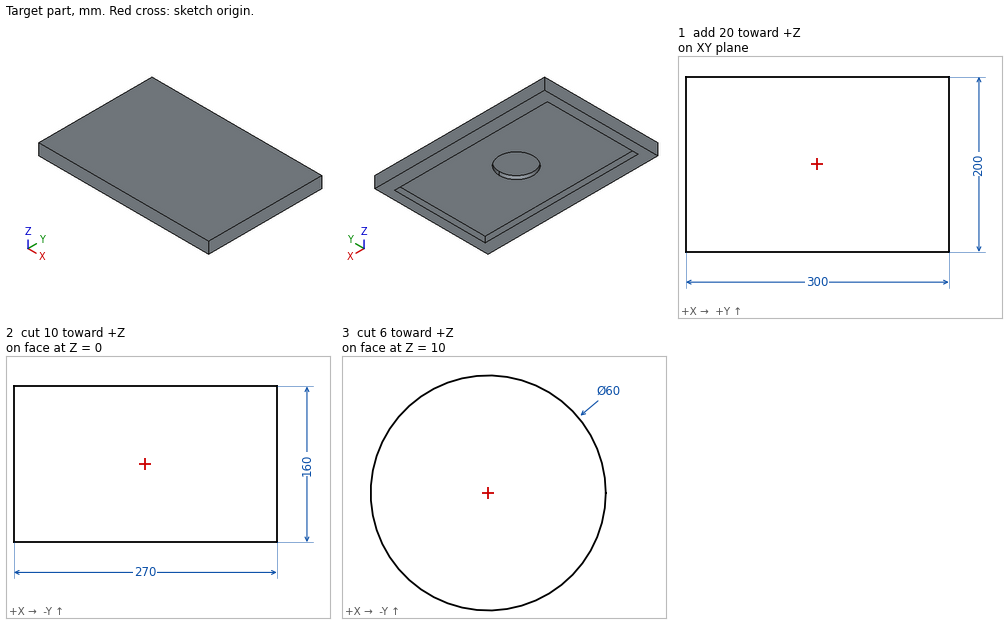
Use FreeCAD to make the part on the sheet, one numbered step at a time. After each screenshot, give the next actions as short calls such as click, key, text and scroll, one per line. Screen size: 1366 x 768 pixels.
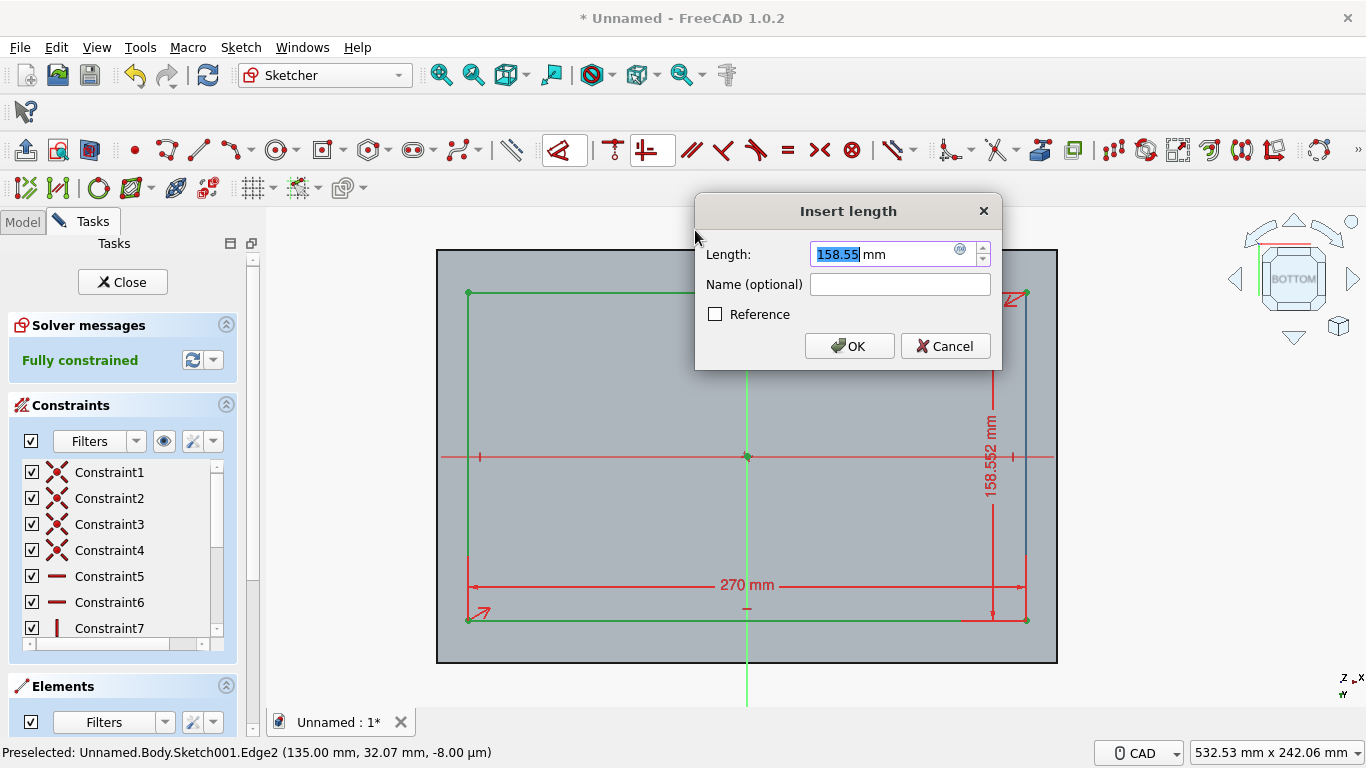
text(160)
key(Return)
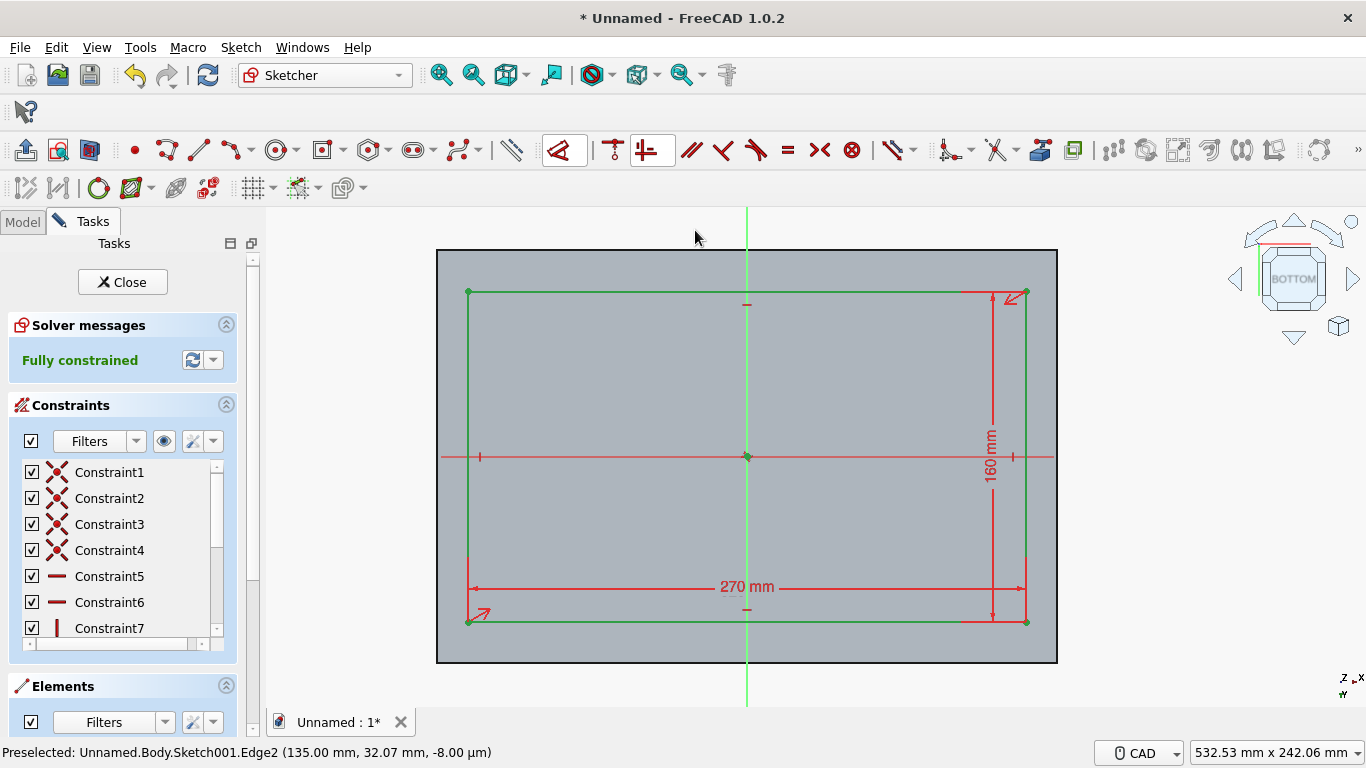
click(123, 282)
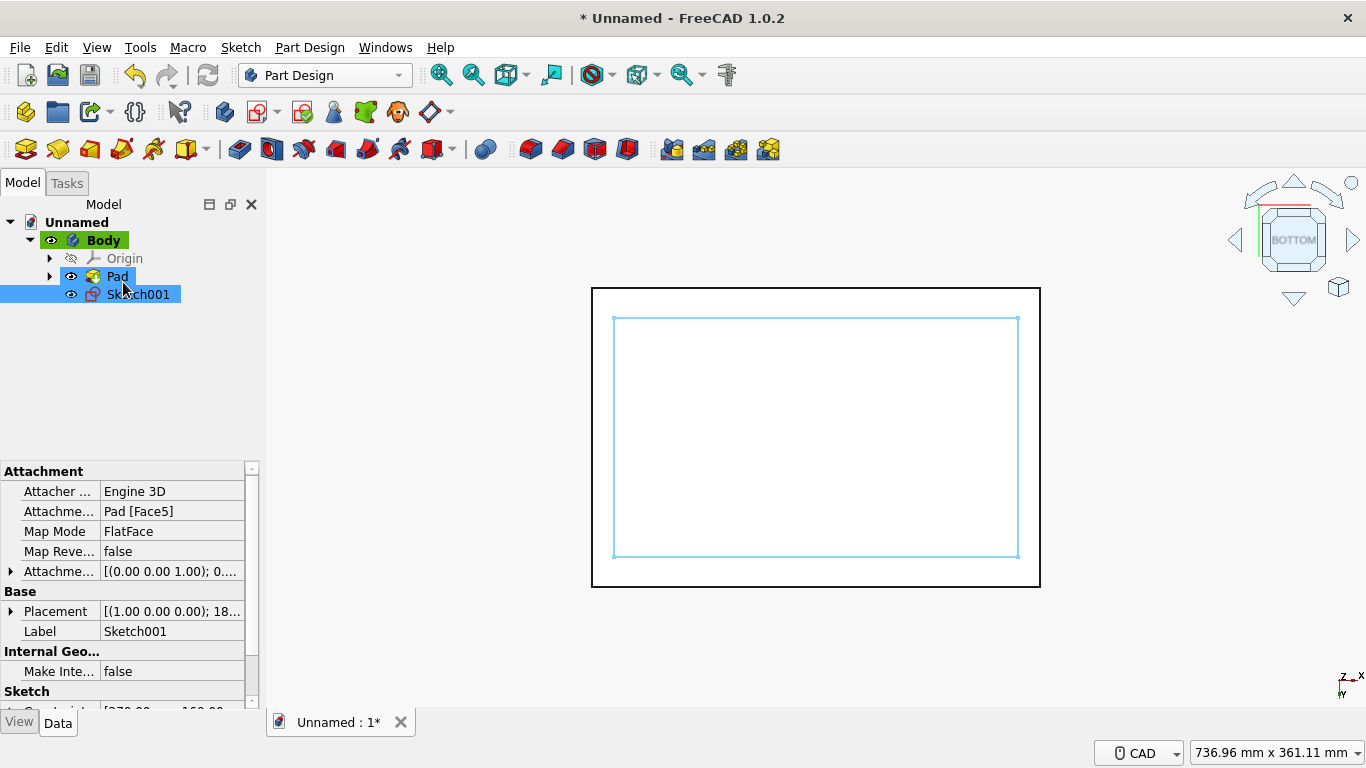
click(240, 150)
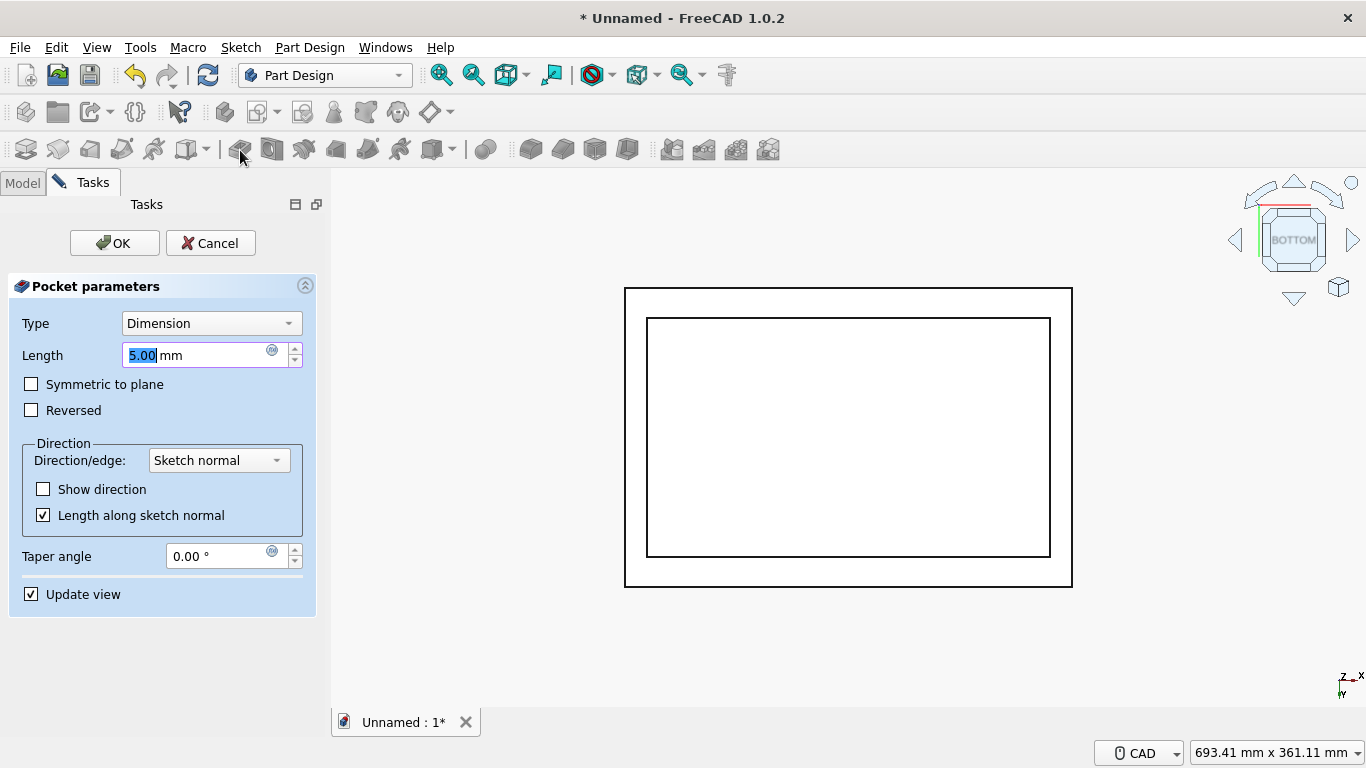
text(10)
key(Tab)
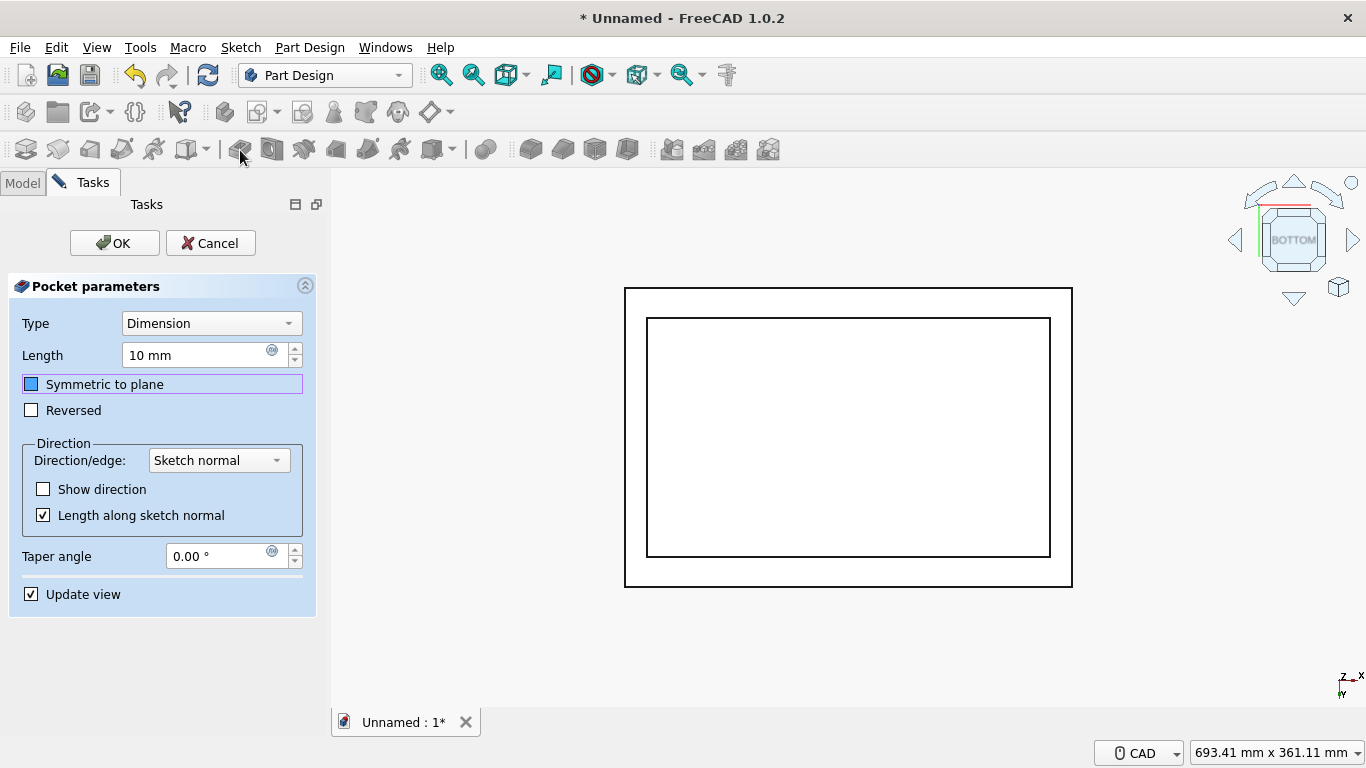
click(115, 243)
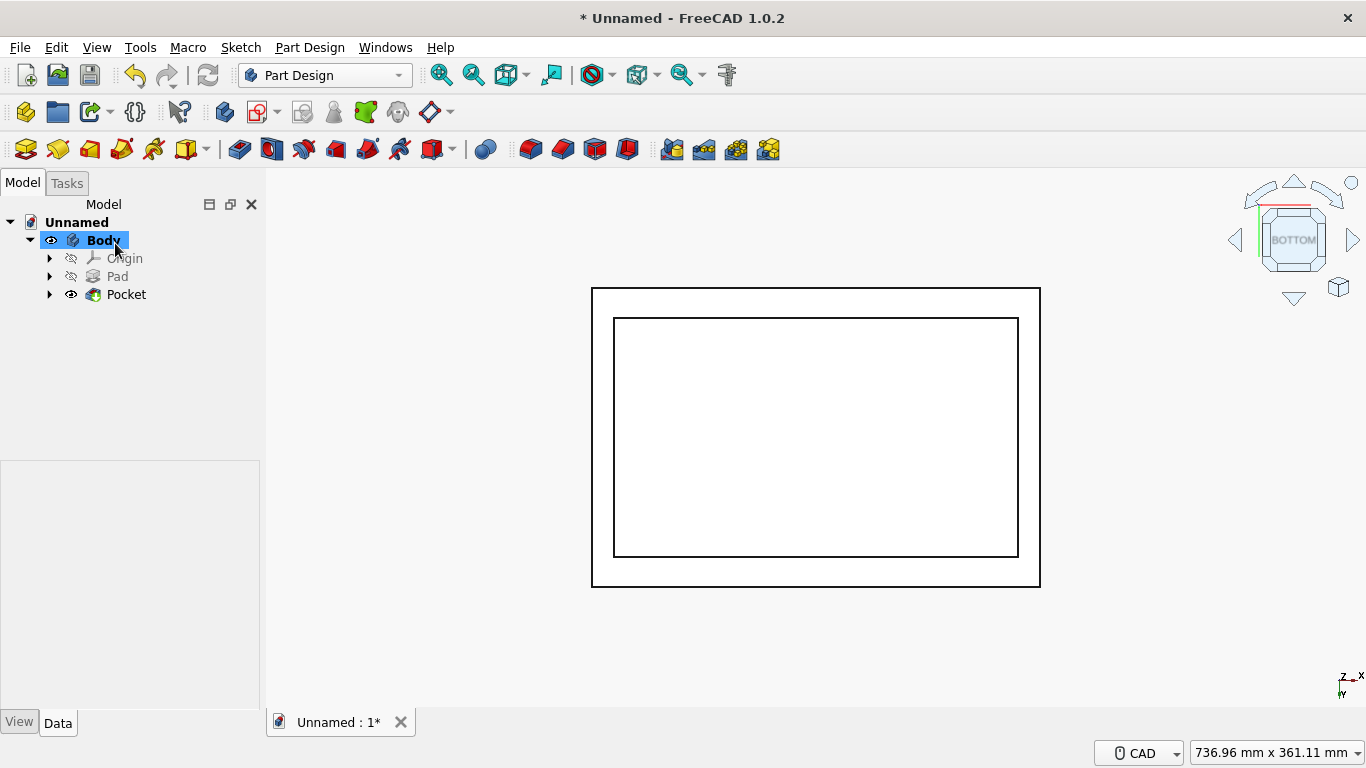
click(874, 437)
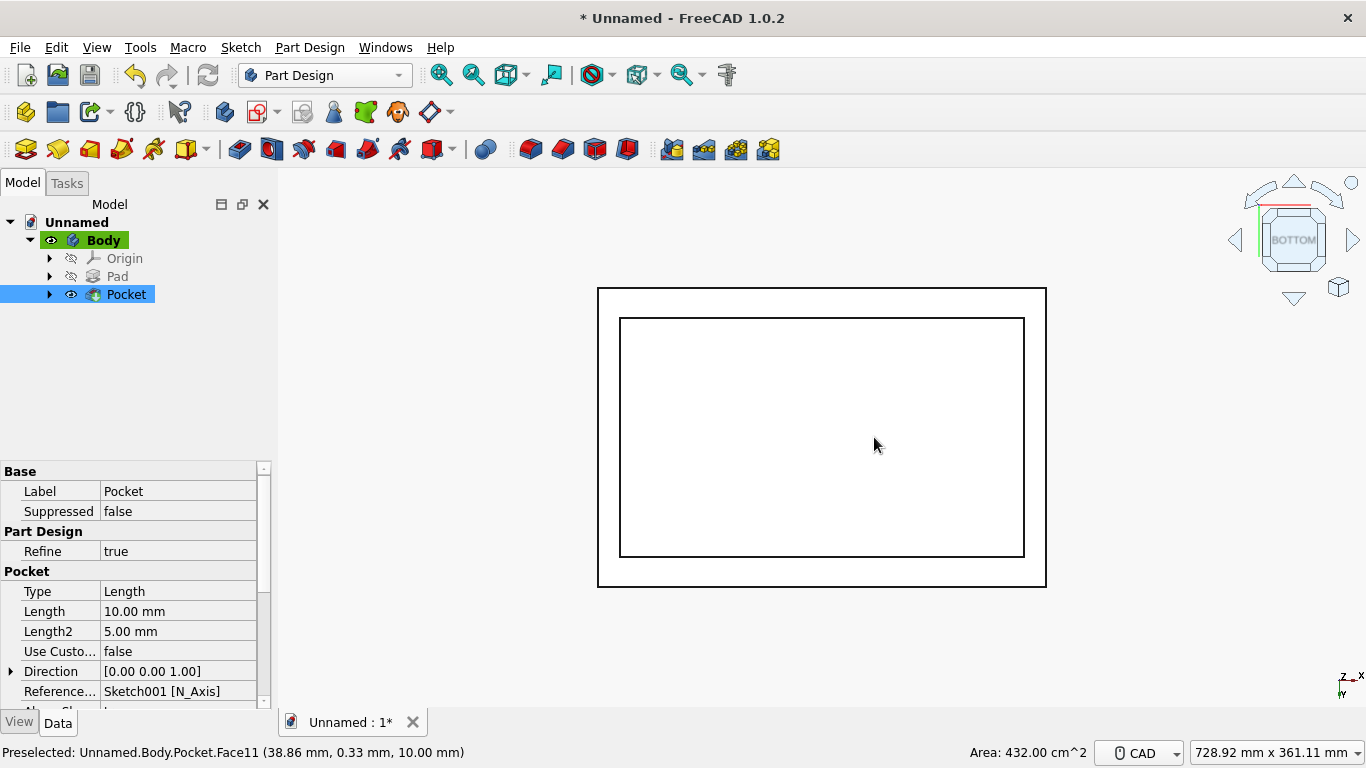
click(258, 112)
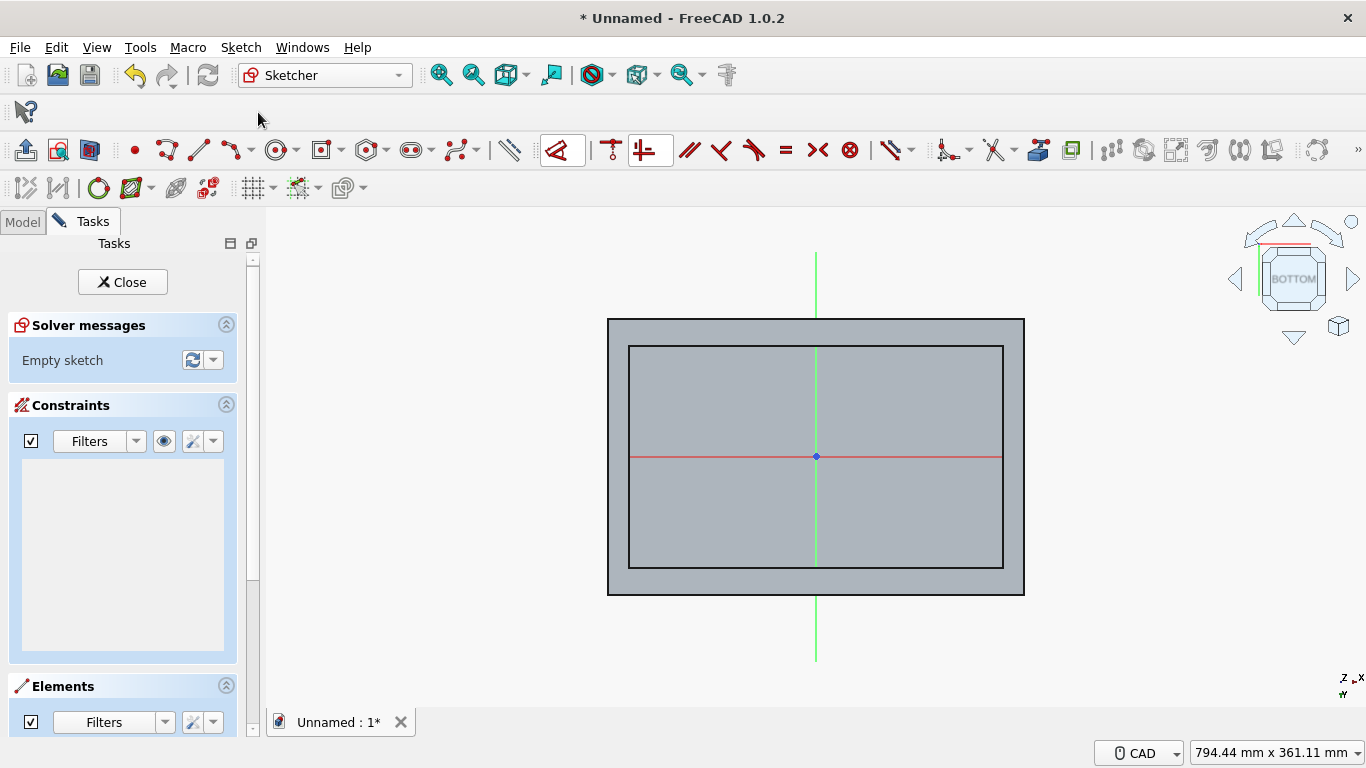
key(q)
key(s)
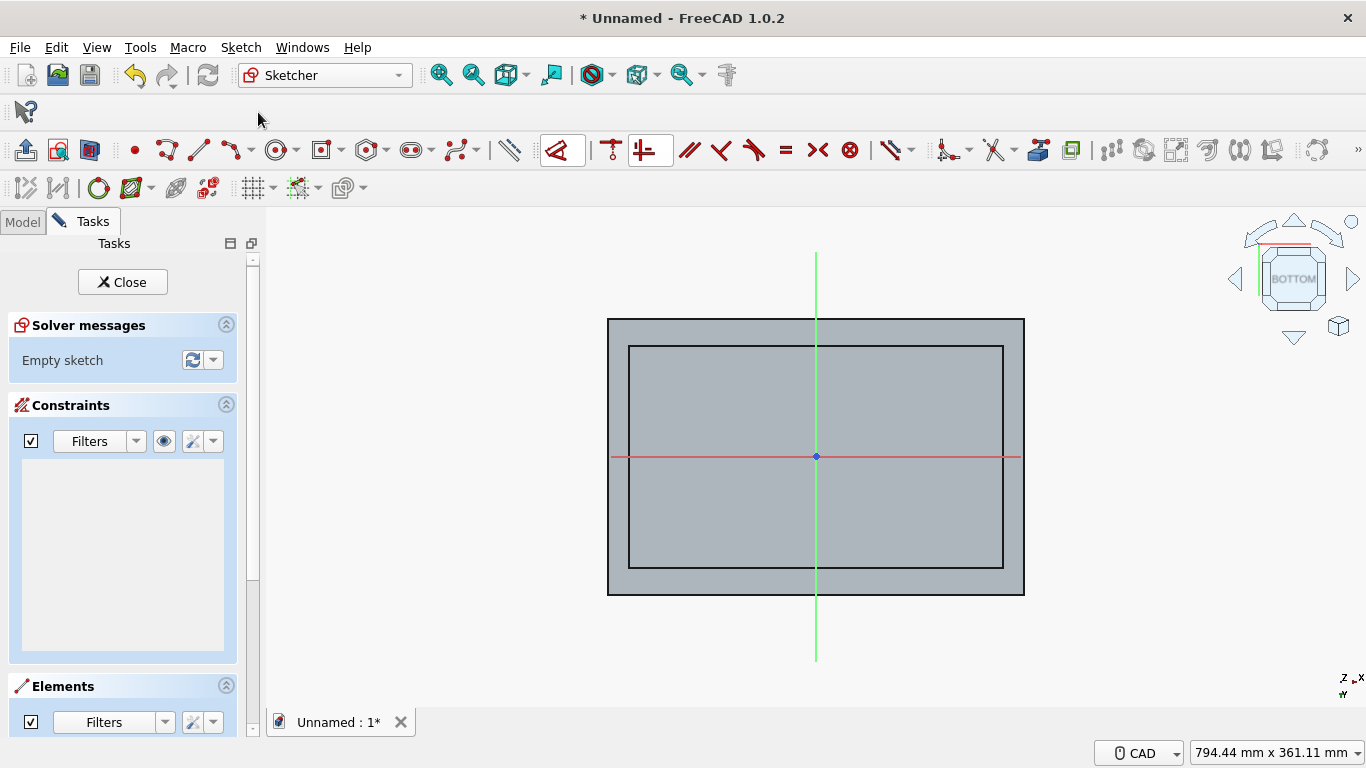
scroll(838, 457, up, 7)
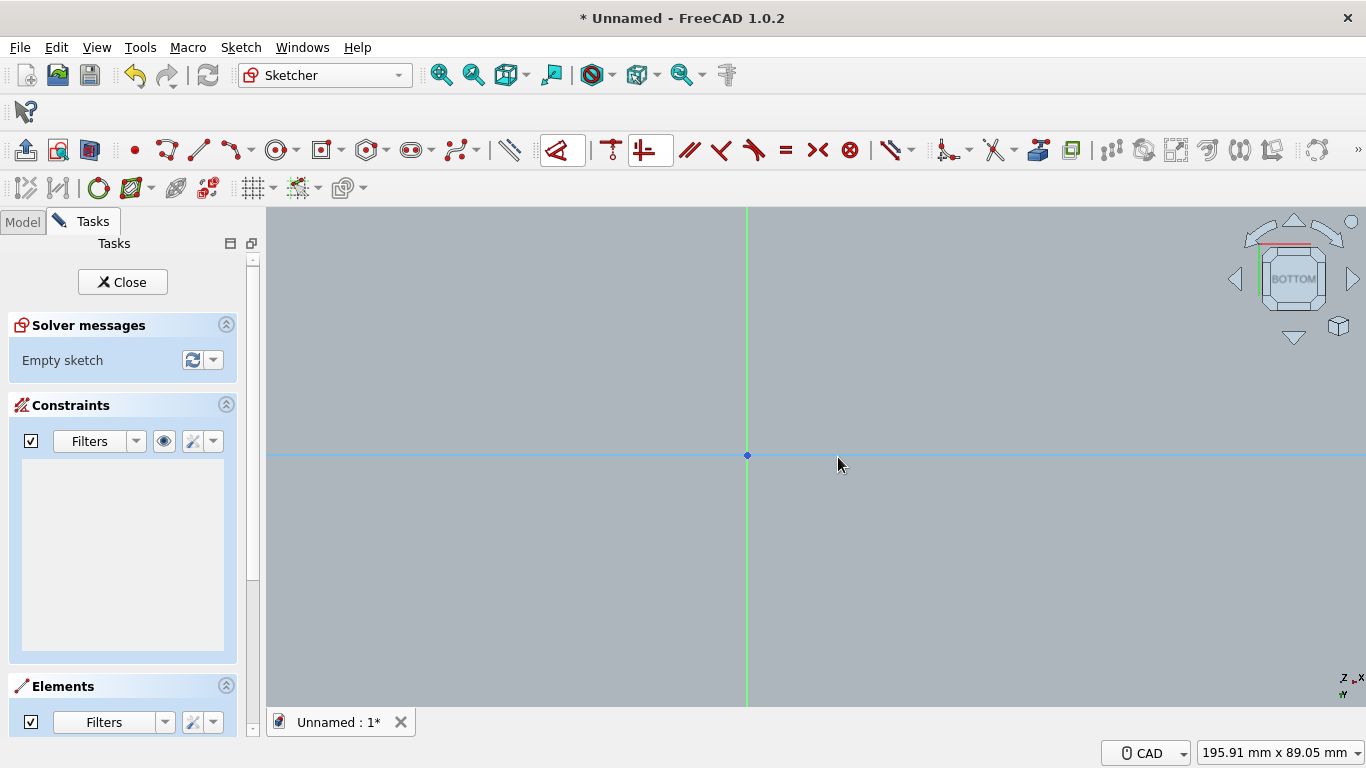
click(276, 150)